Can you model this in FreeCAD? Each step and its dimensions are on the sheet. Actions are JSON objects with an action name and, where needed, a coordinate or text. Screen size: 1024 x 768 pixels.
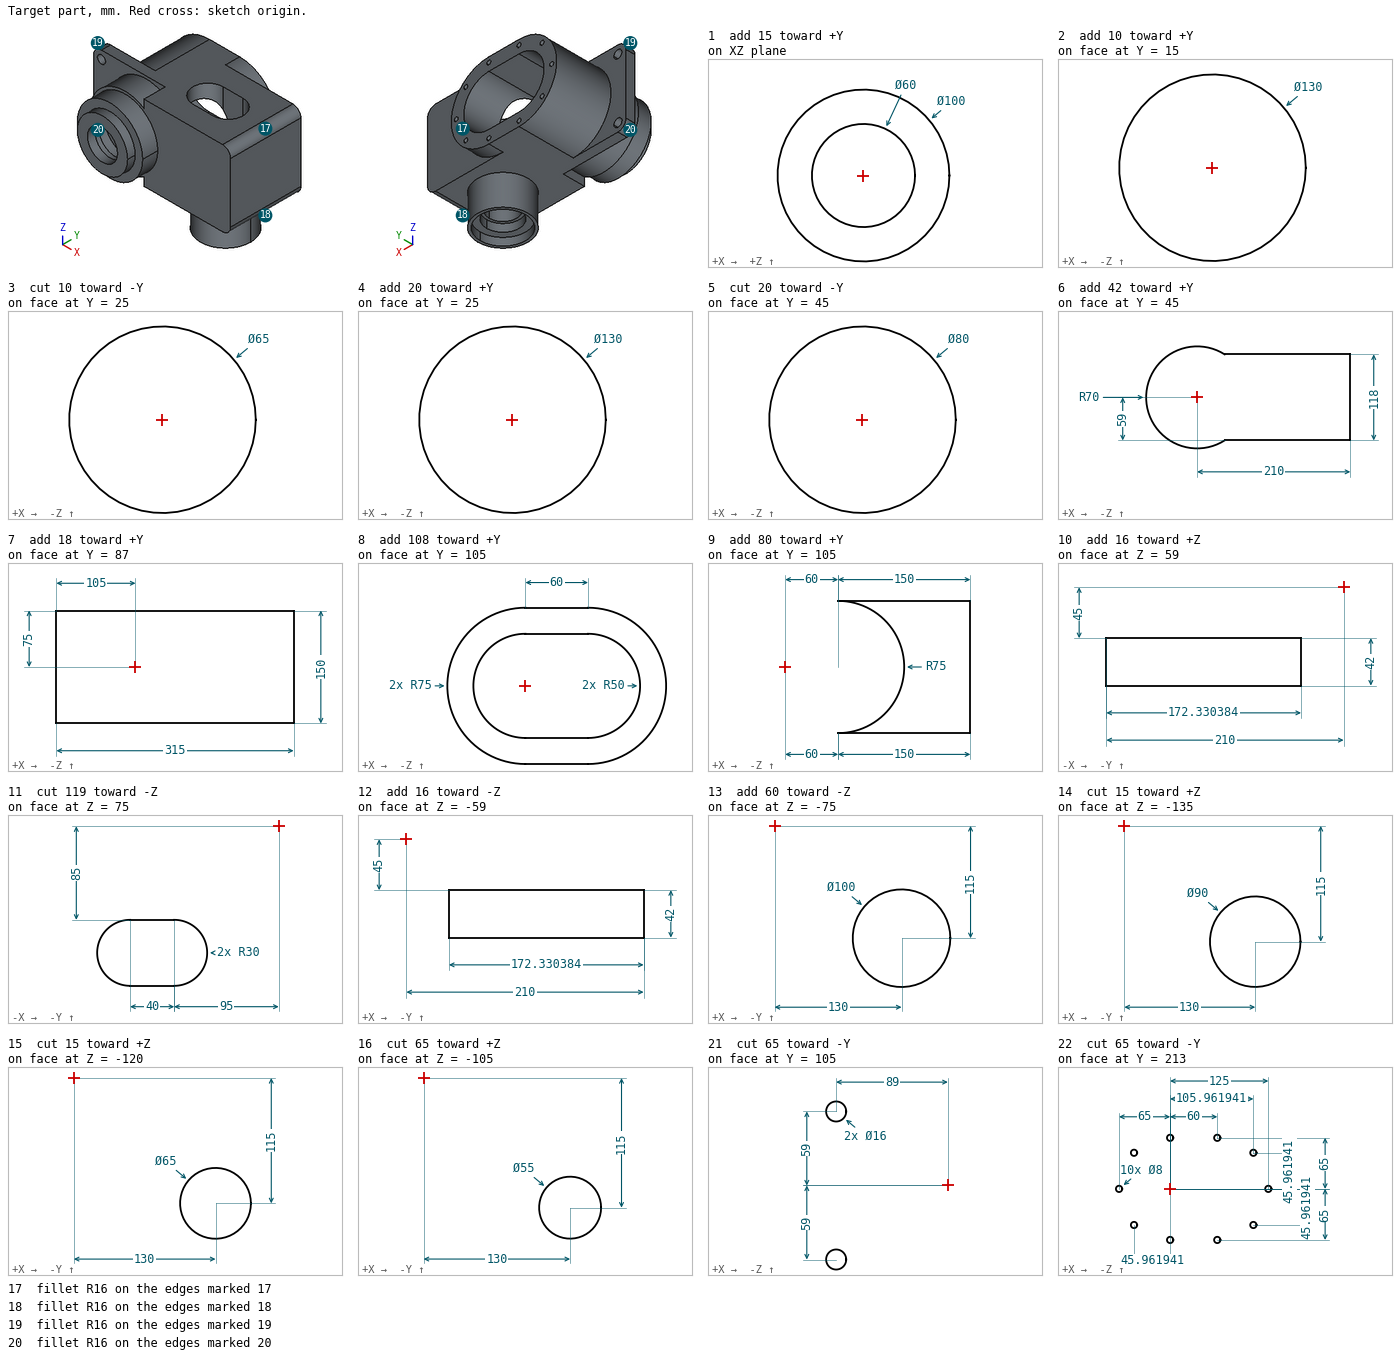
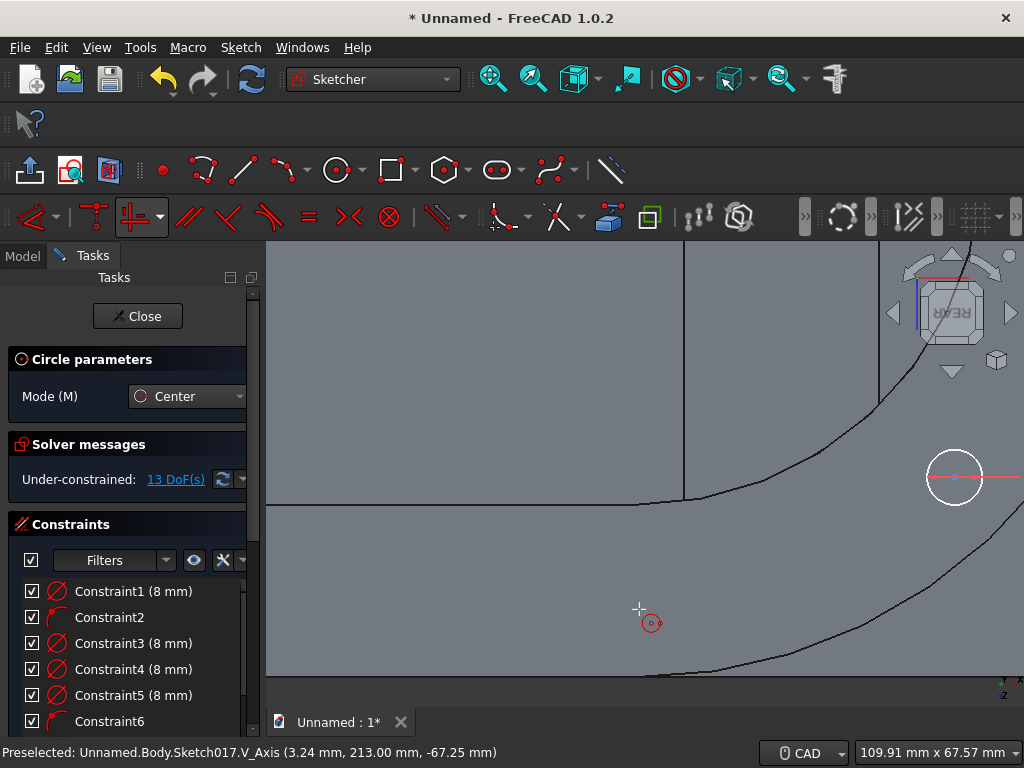
{"action": "left_click", "coordinate": [637, 608]}
{"action": "mouse_move", "coordinate": [657, 589]}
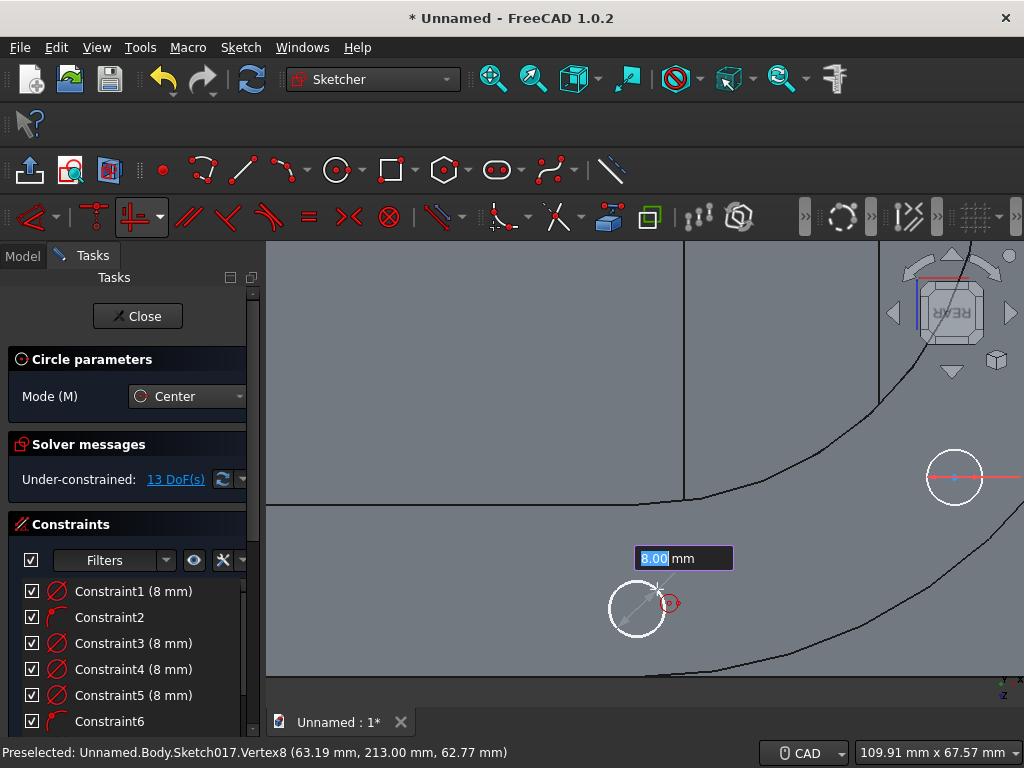
{"action": "type", "text": "8"}
{"action": "key", "text": "Return"}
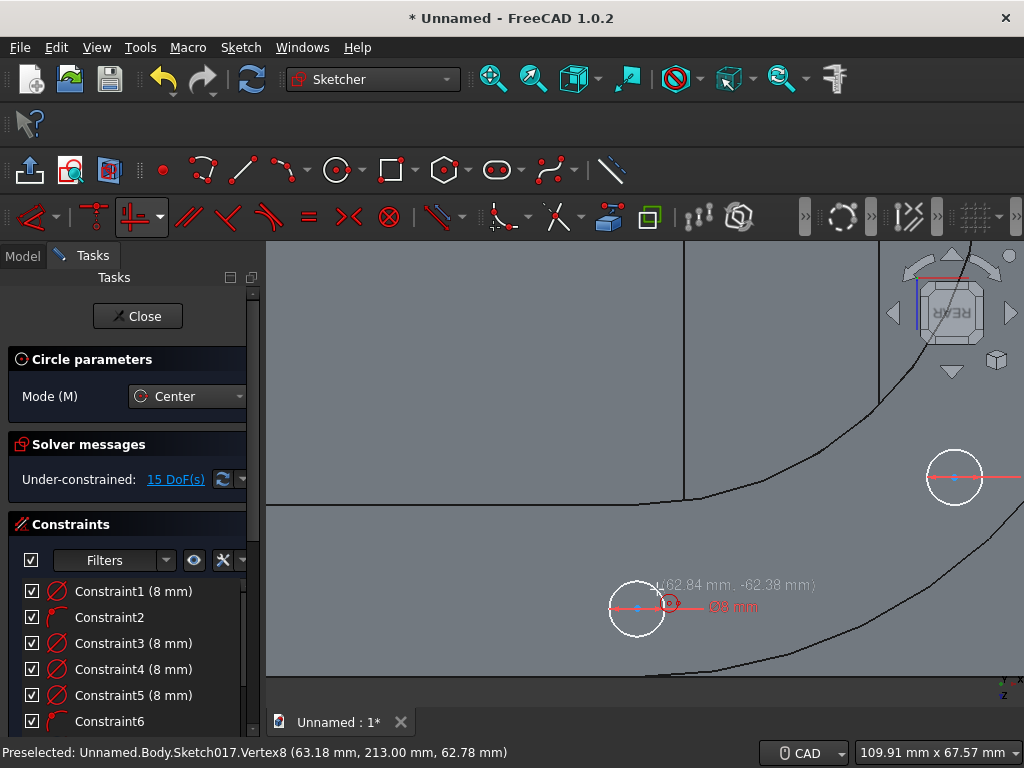
{"action": "scroll", "coordinate": [639, 609], "scroll_direction": "down", "scroll_amount": 6}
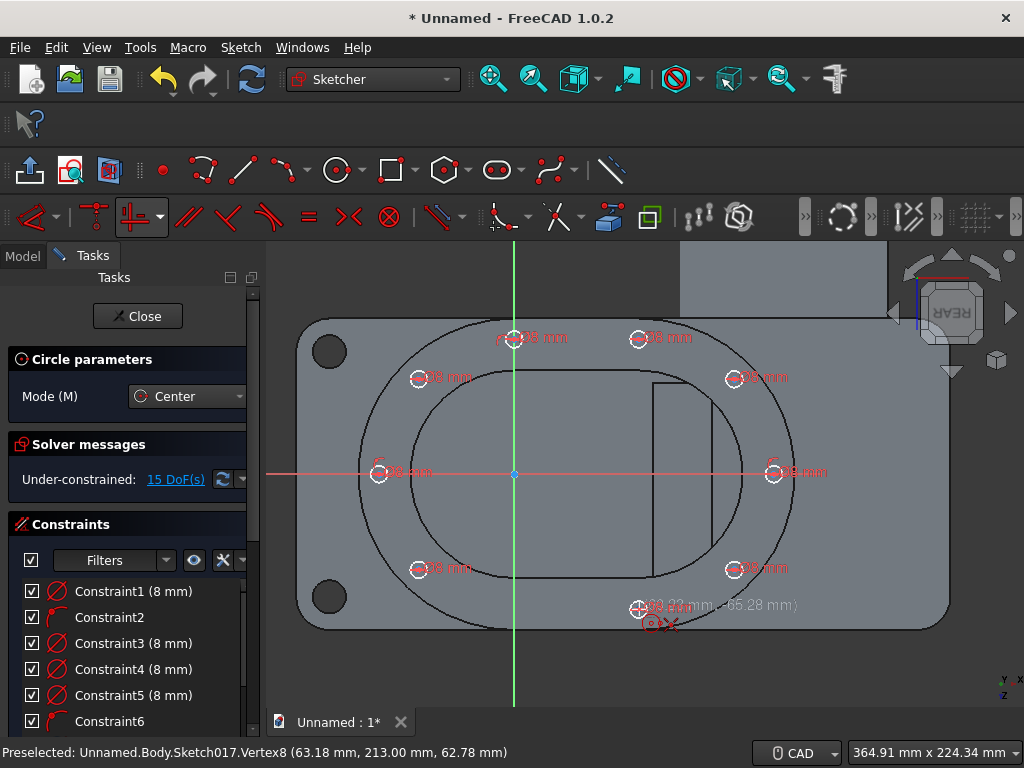
{"action": "scroll", "coordinate": [514, 609], "scroll_direction": "up", "scroll_amount": 6}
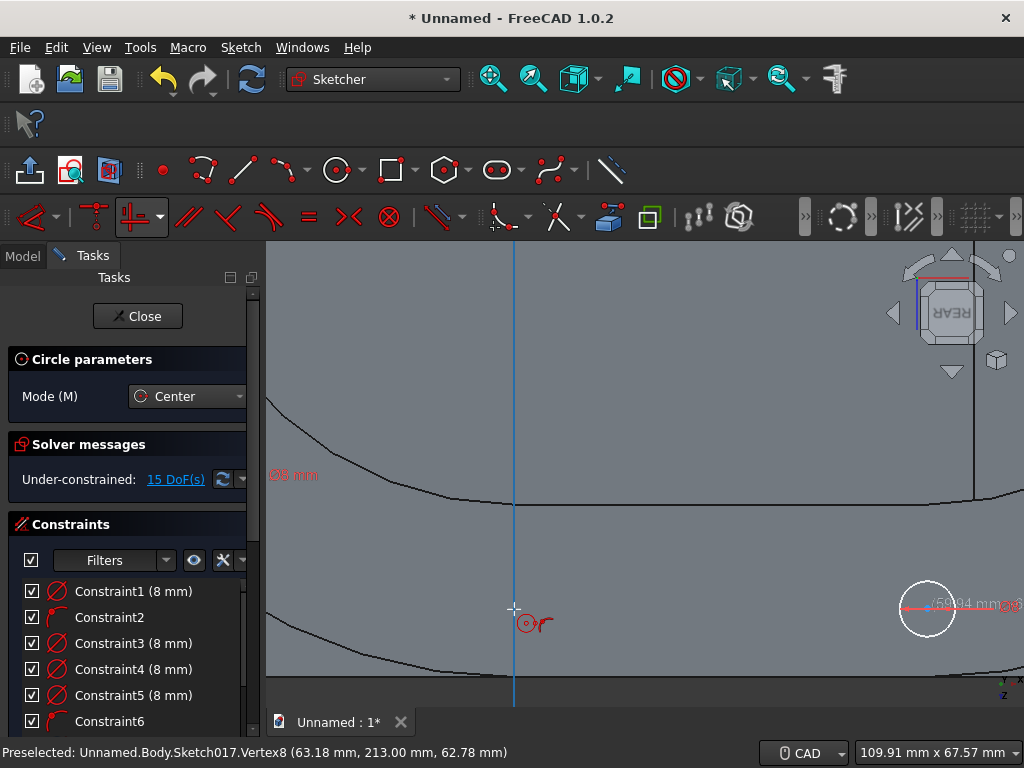
{"action": "left_click", "coordinate": [514, 608]}
{"action": "mouse_move", "coordinate": [533, 589]}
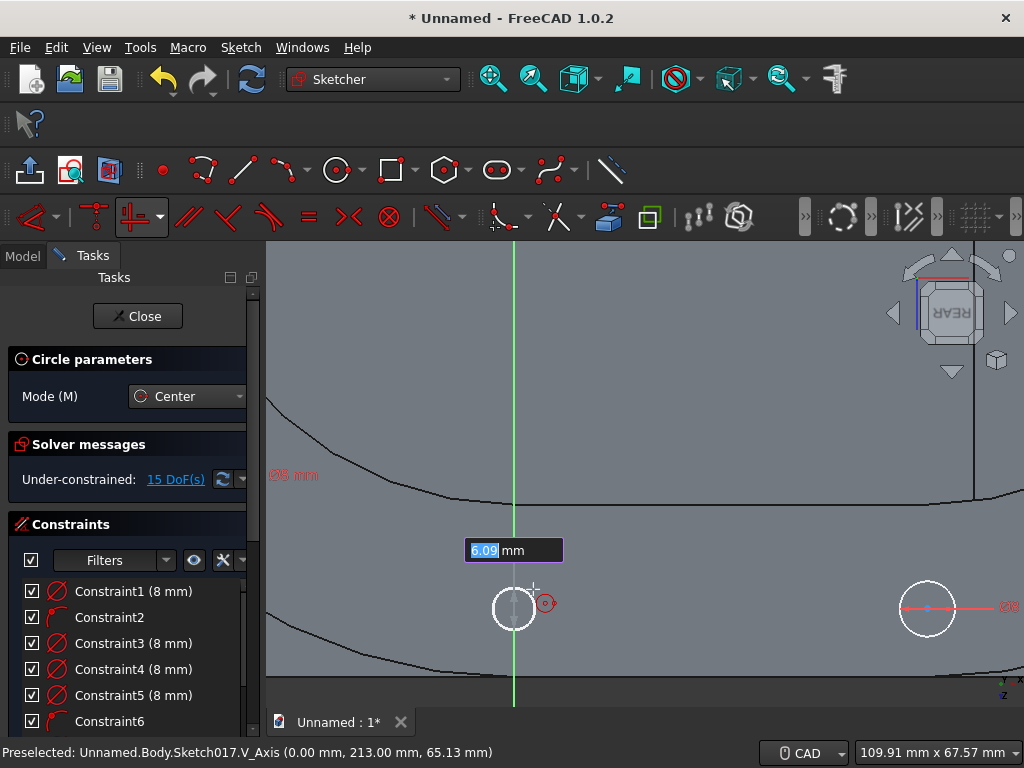
{"action": "type", "text": "8"}
{"action": "key", "text": "Return"}
{"action": "key", "text": "Escape"}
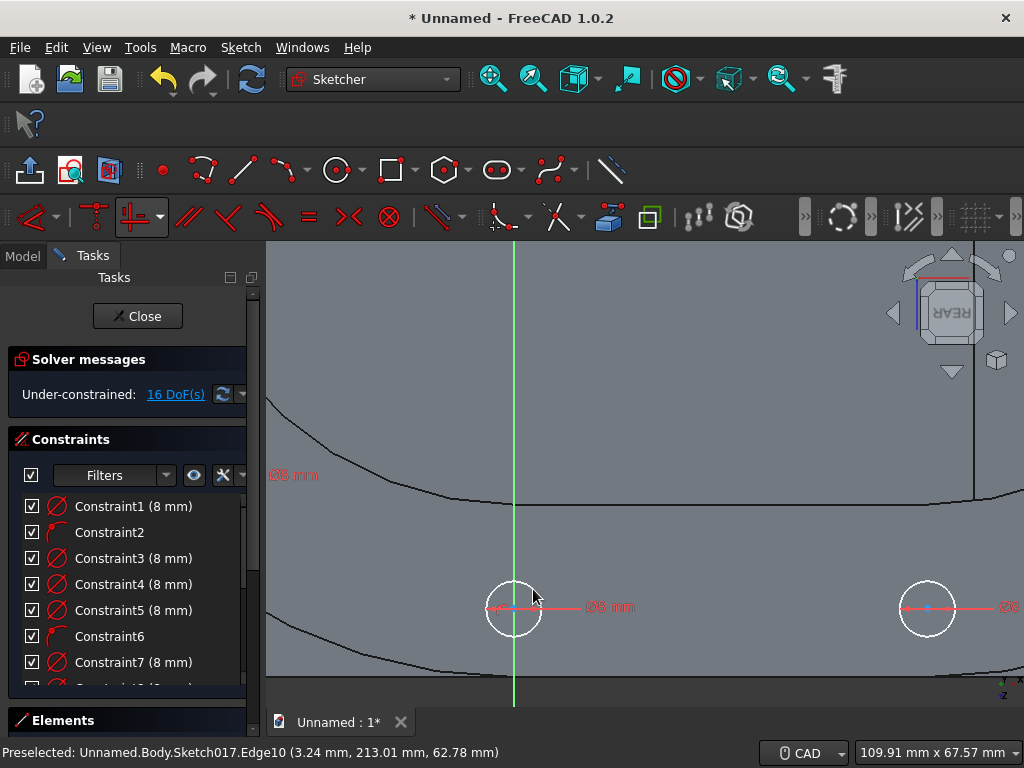
{"action": "scroll", "coordinate": [514, 609], "scroll_direction": "down", "scroll_amount": 6}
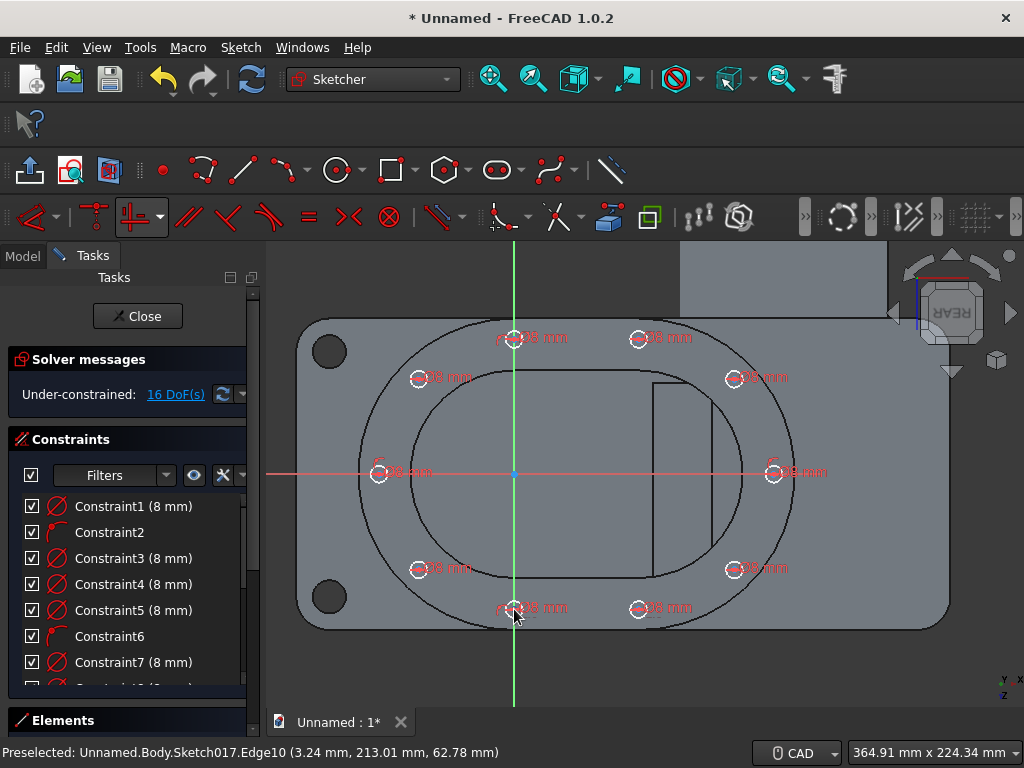
{"action": "left_click", "coordinate": [734, 379]}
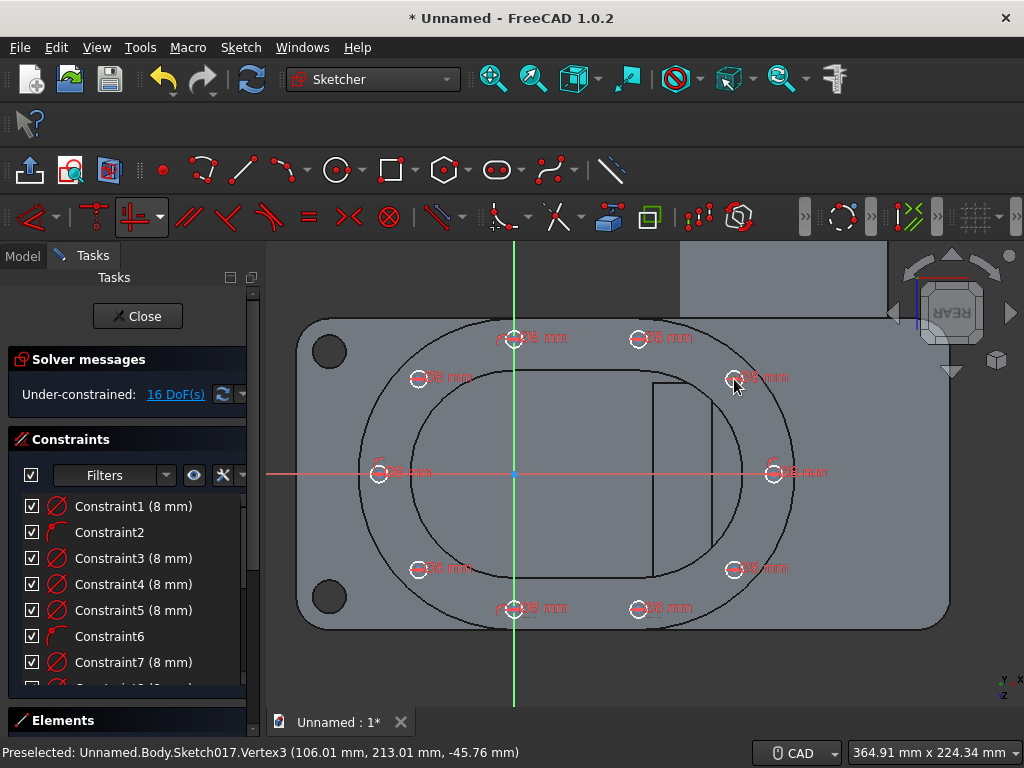
{"action": "left_click", "coordinate": [734, 570]}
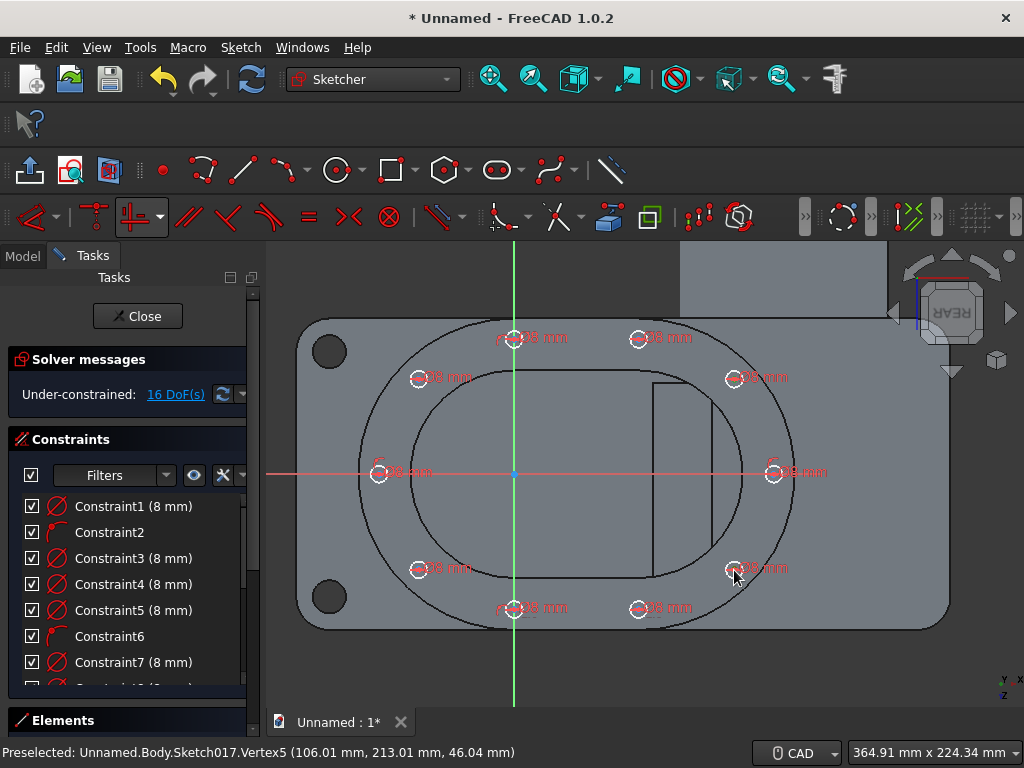
{"action": "key", "text": "v"}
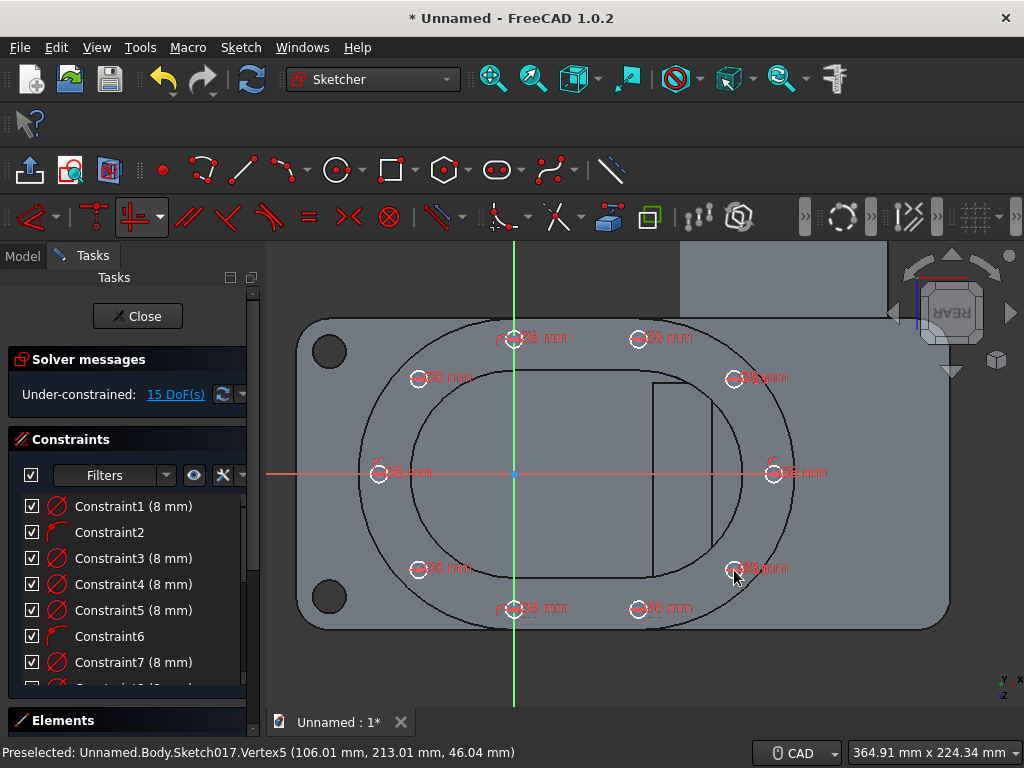
{"action": "left_click", "coordinate": [734, 570]}